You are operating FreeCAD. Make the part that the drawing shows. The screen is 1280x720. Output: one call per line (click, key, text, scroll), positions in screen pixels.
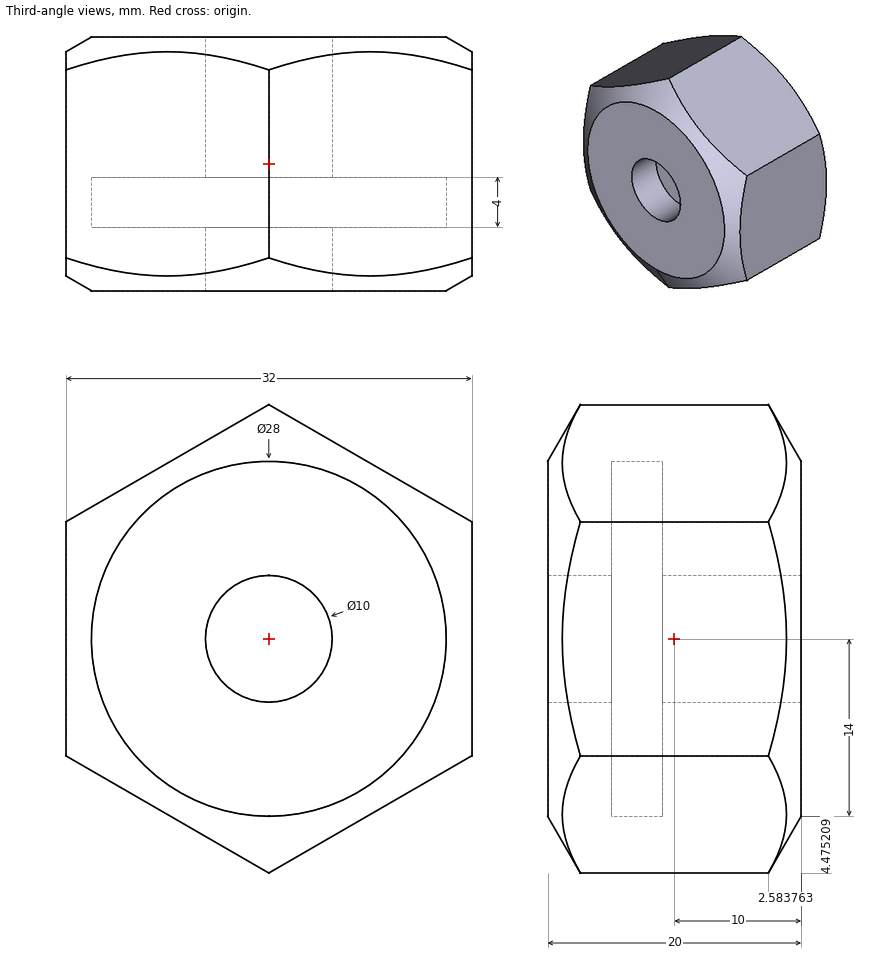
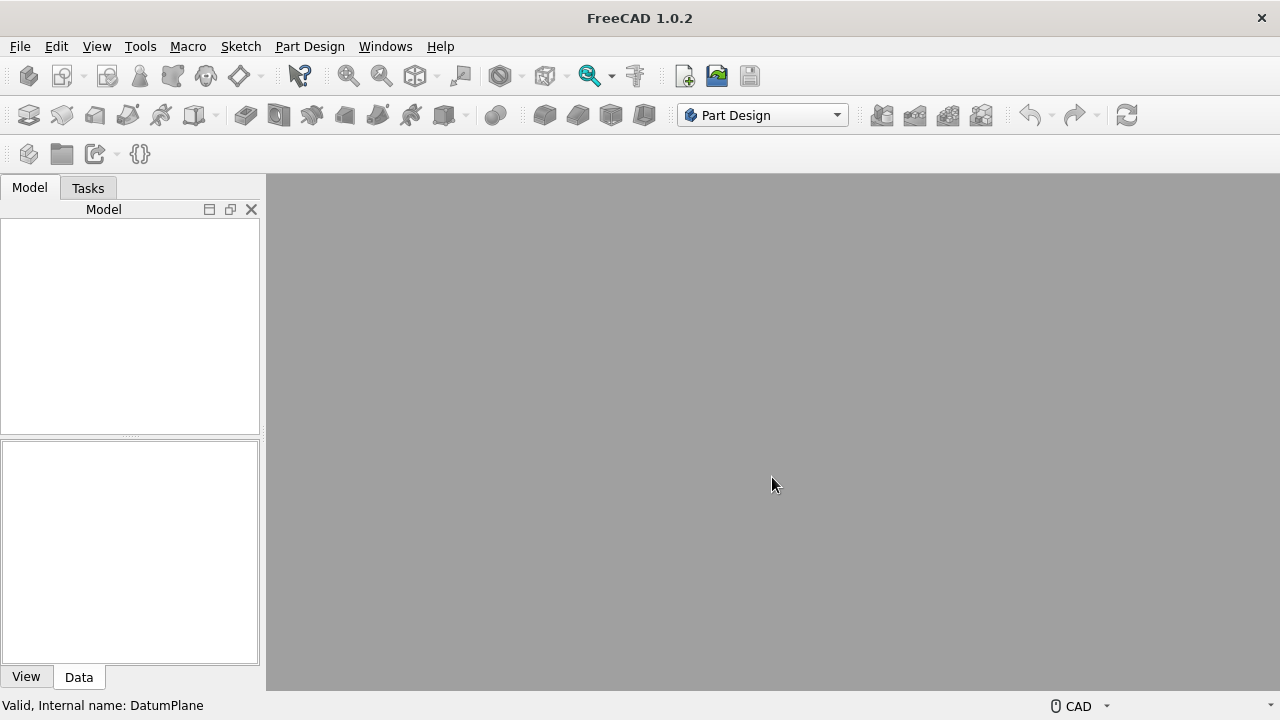
click(684, 76)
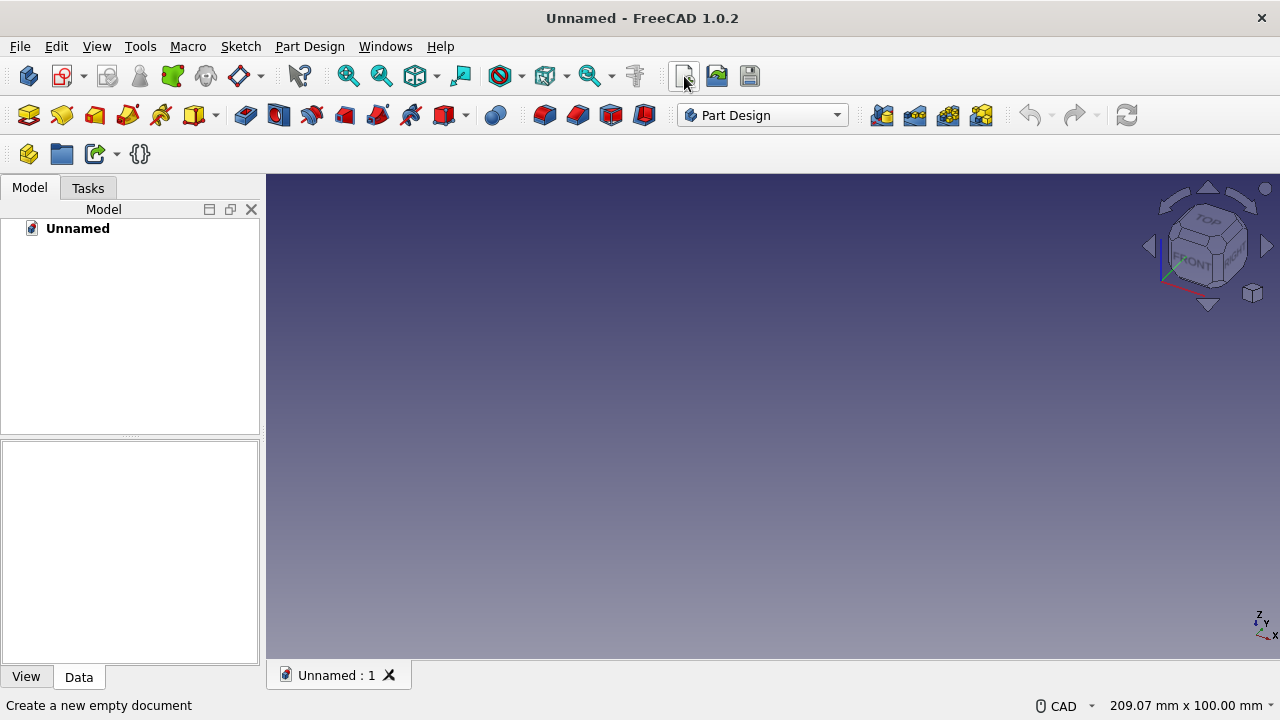
click(62, 76)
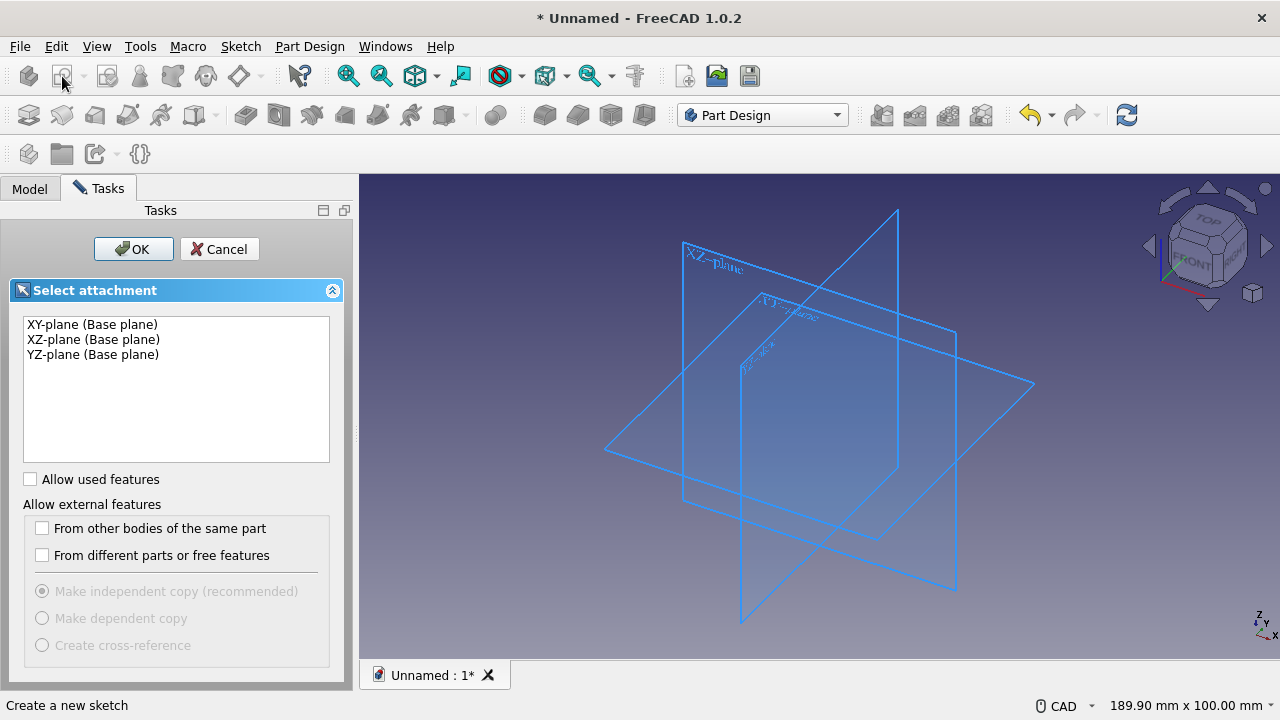
click(84, 340)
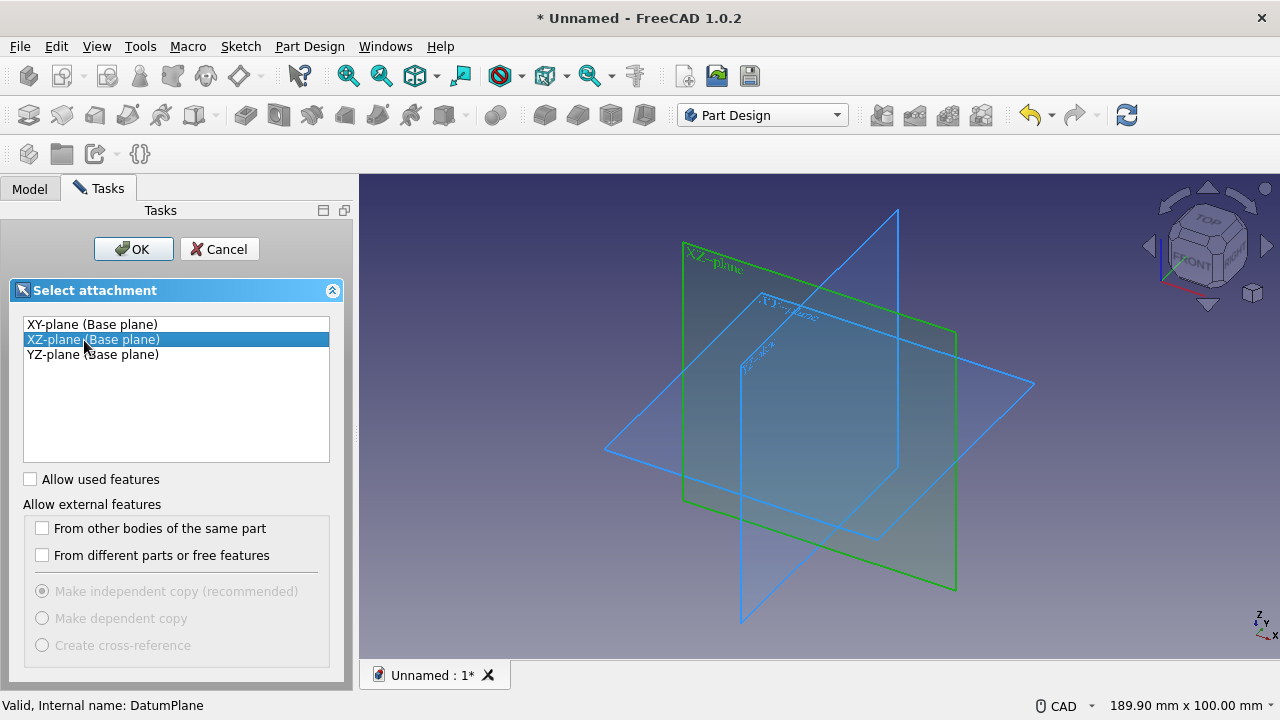
click(134, 249)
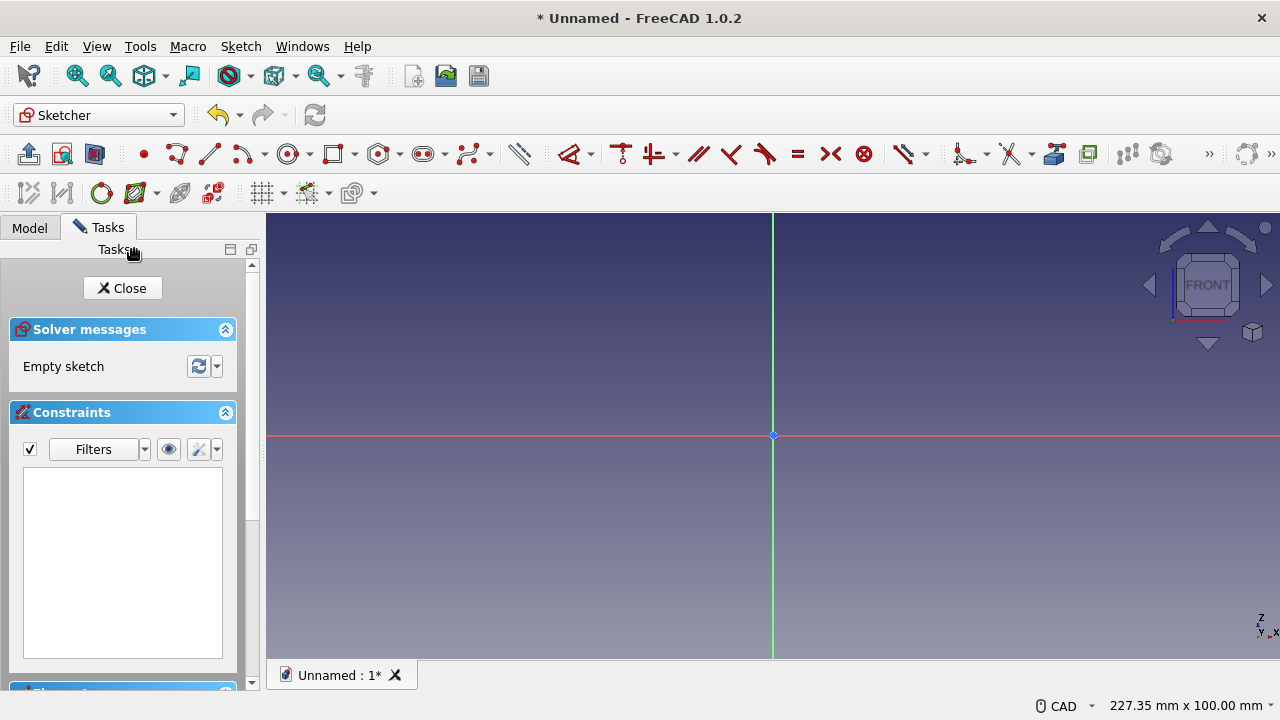
scroll(856, 436, up, 3)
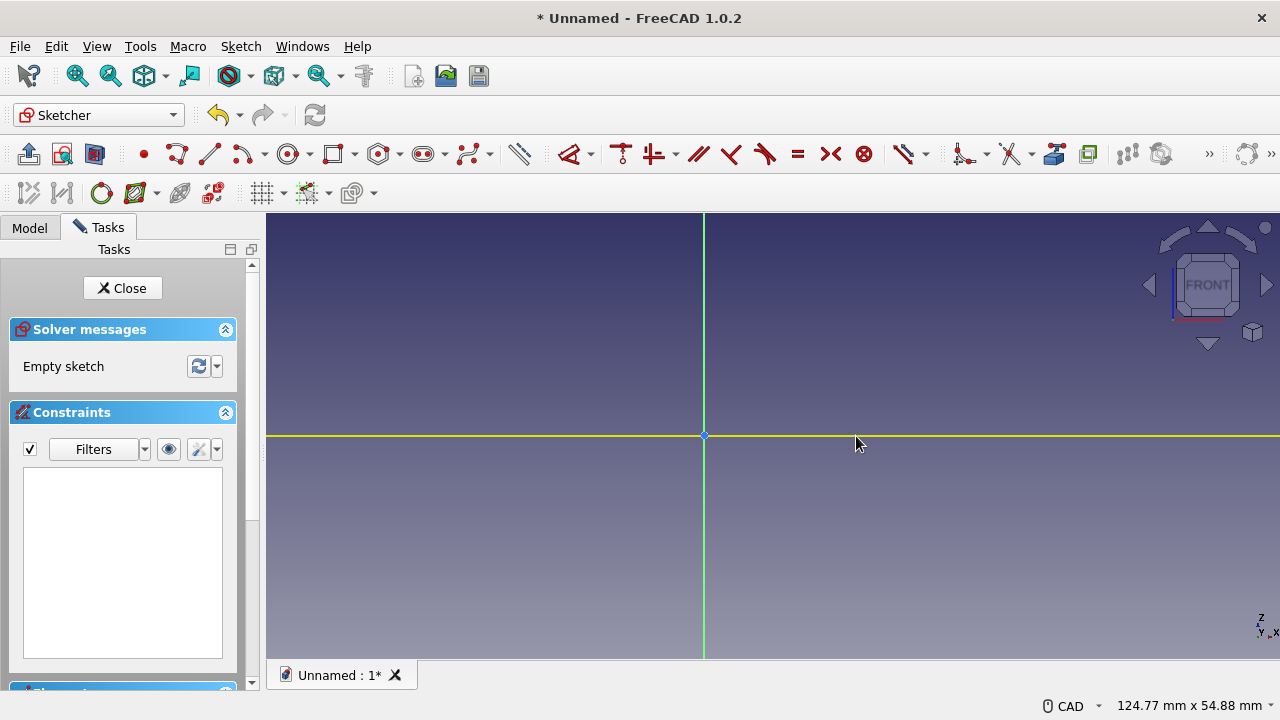
click(378, 154)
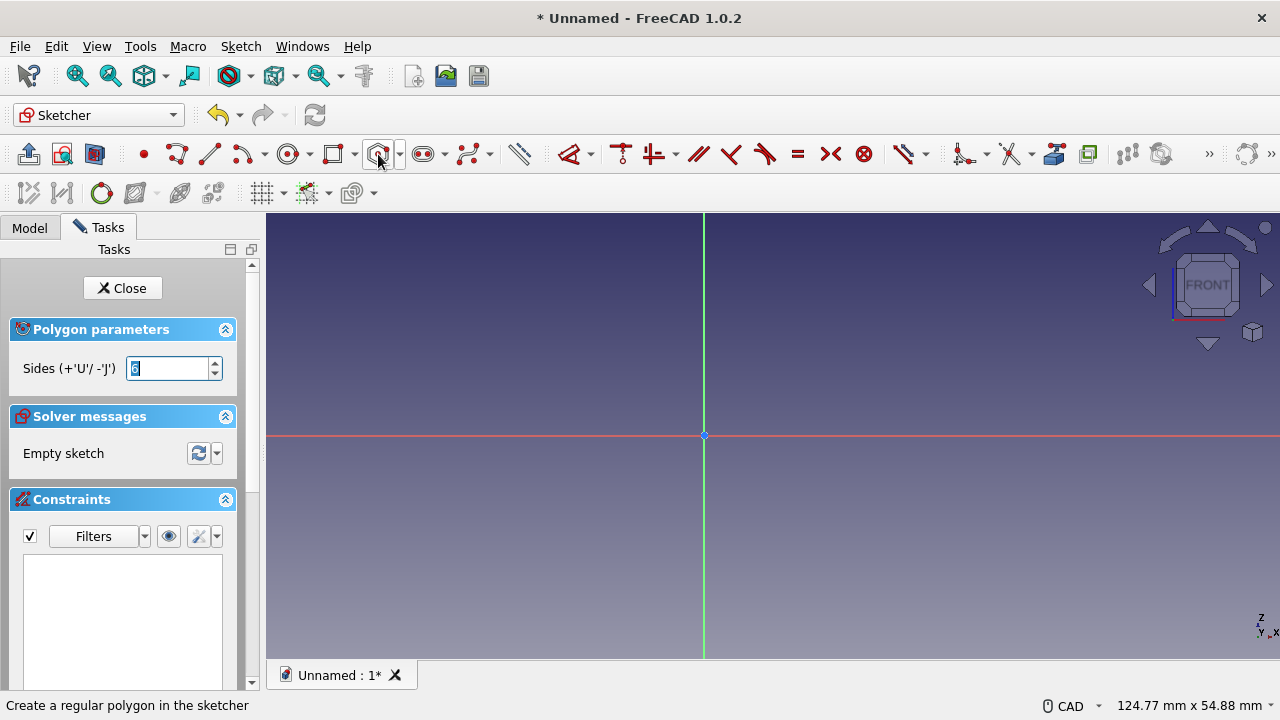
click(704, 436)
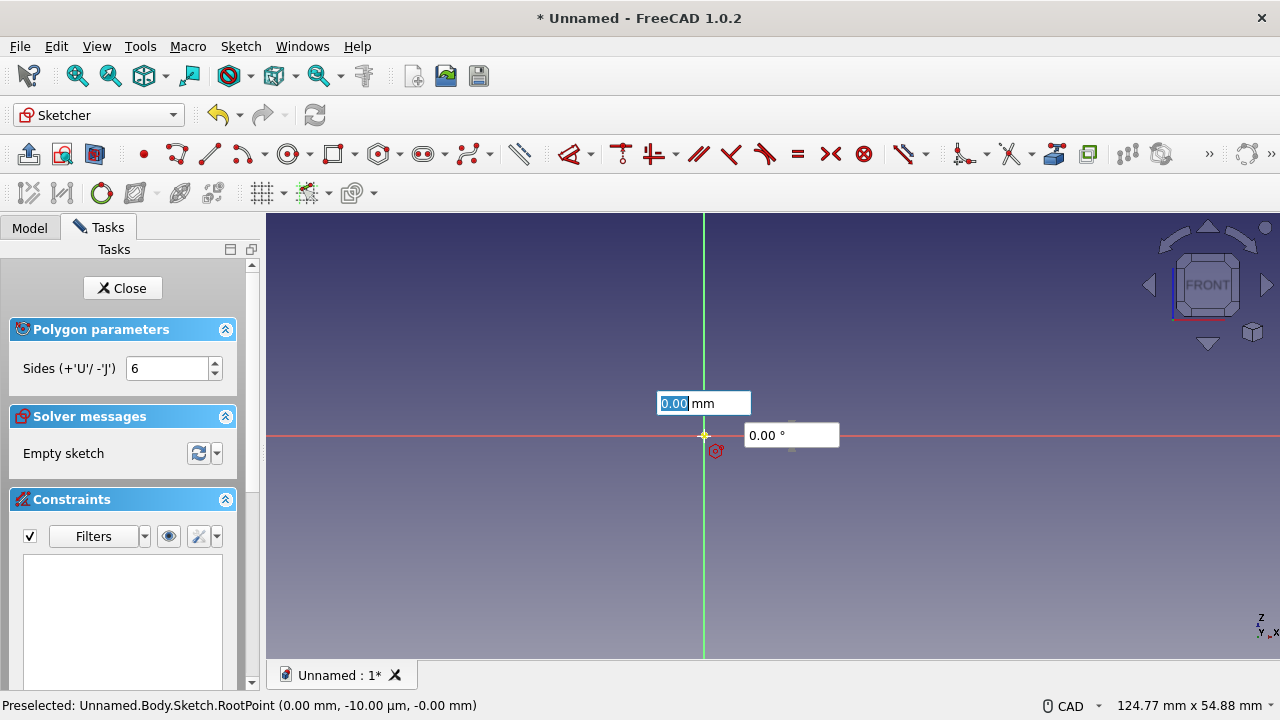
click(704, 586)
right_click(704, 586)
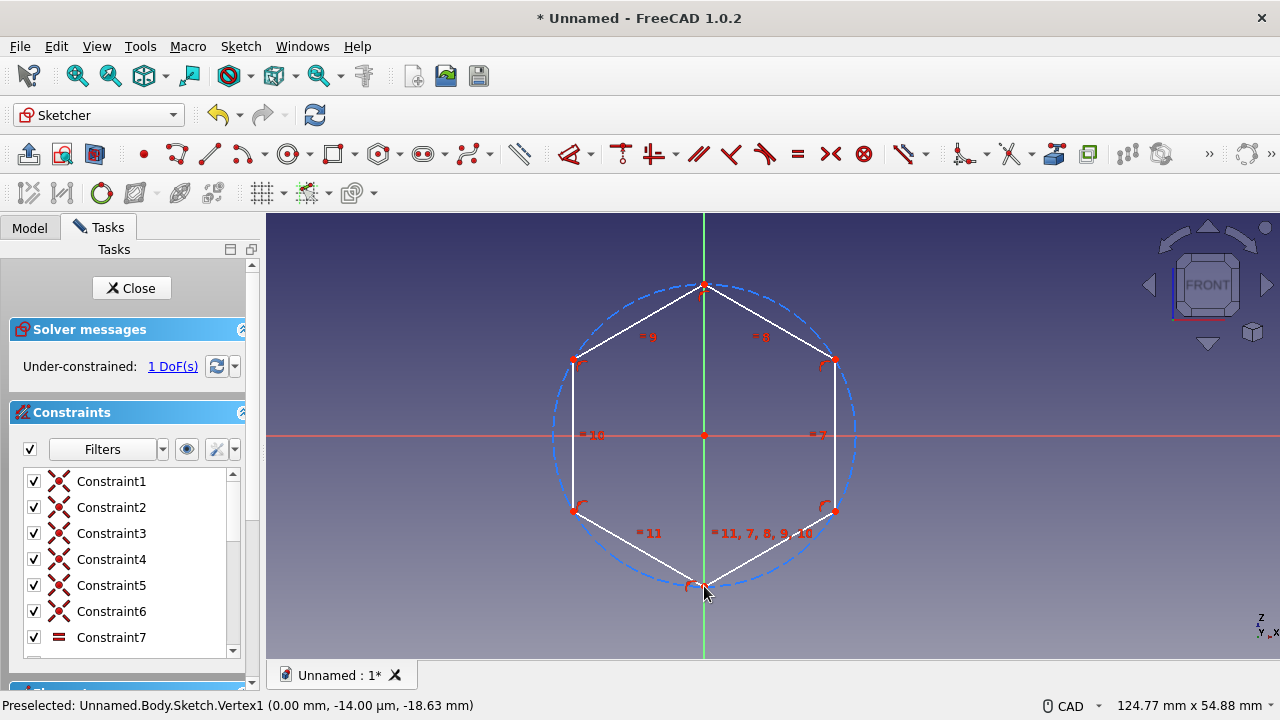
click(573, 360)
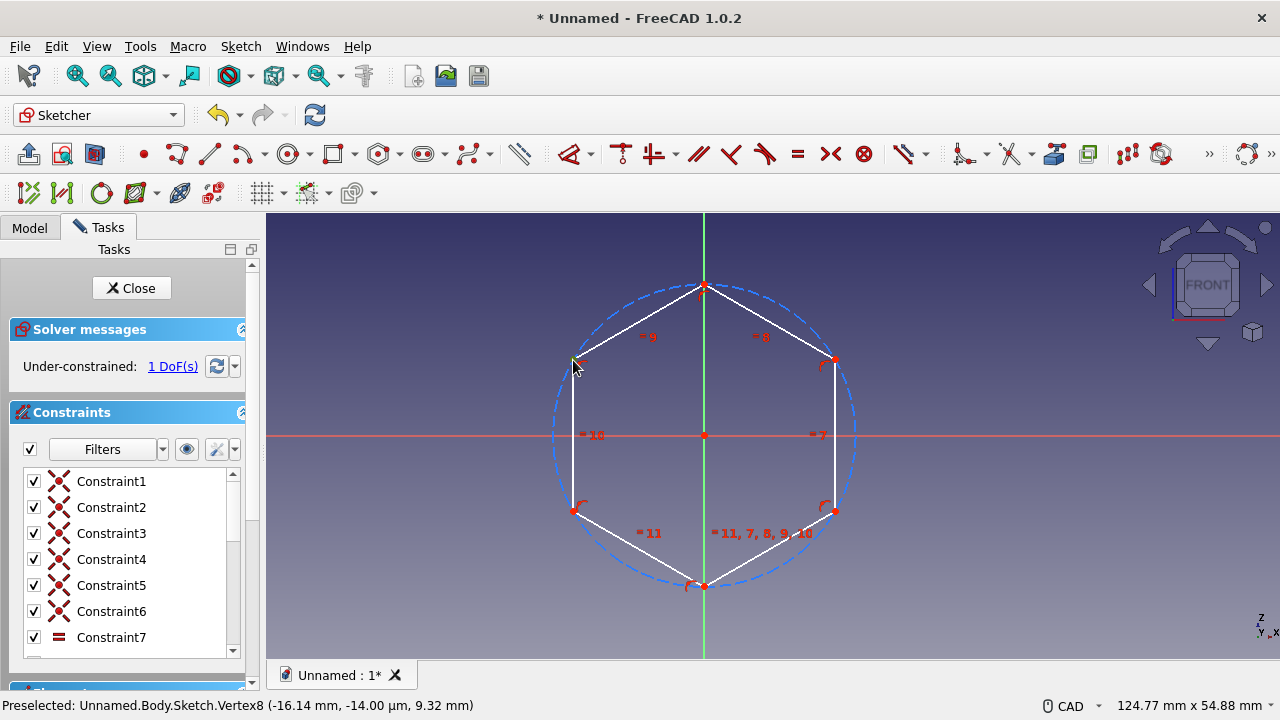
click(835, 511)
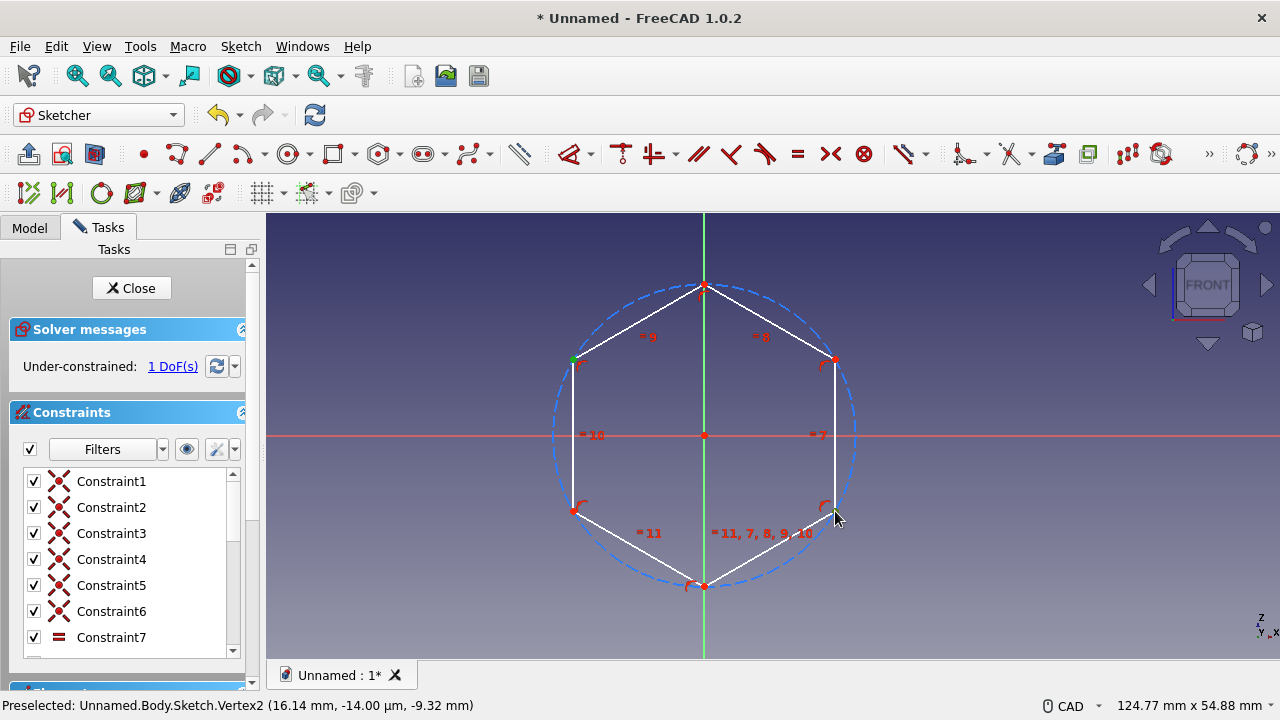
click(590, 154)